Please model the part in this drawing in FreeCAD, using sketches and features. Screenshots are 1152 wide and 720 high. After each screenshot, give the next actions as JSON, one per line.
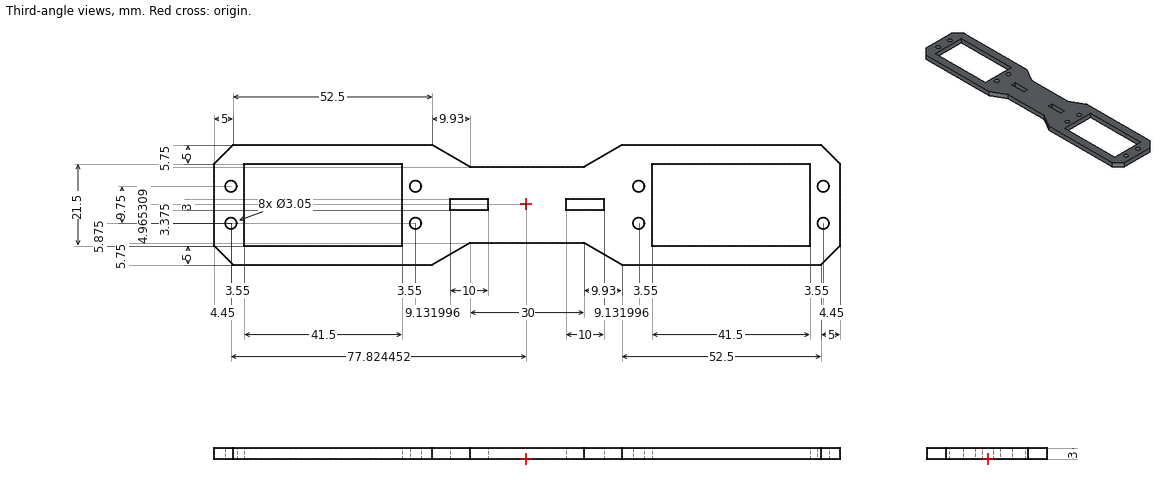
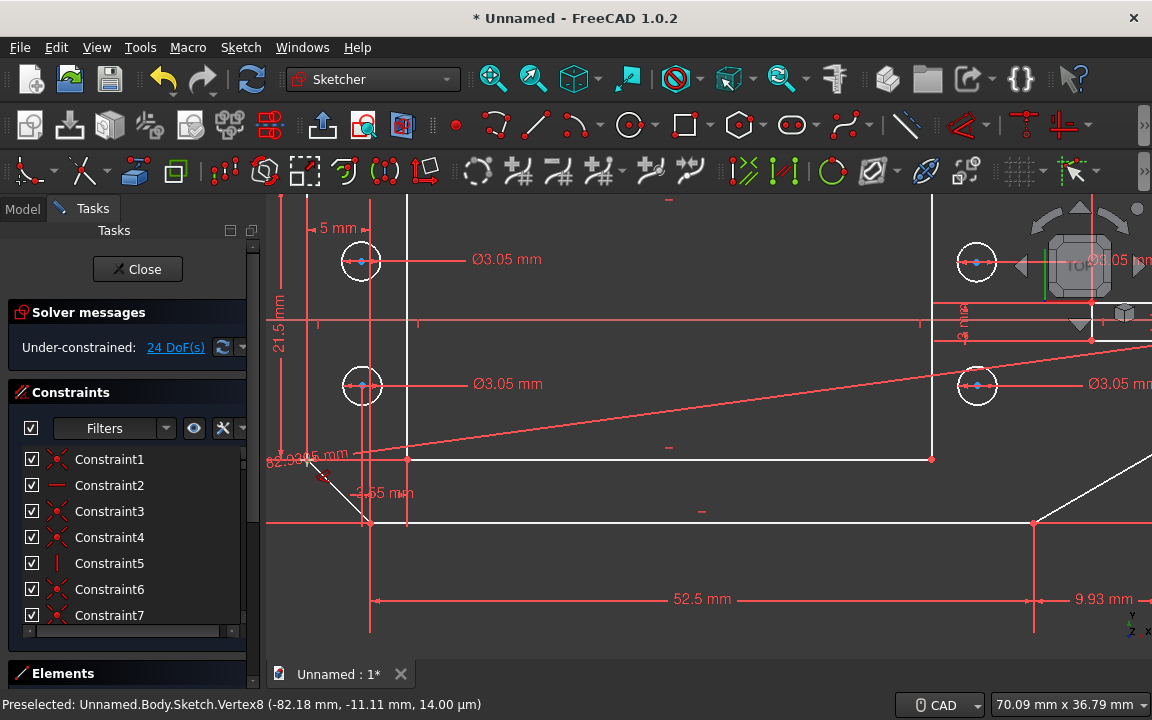
{"action": "left_click", "coordinate": [362, 386]}
{"action": "left_click", "coordinate": [335, 352]}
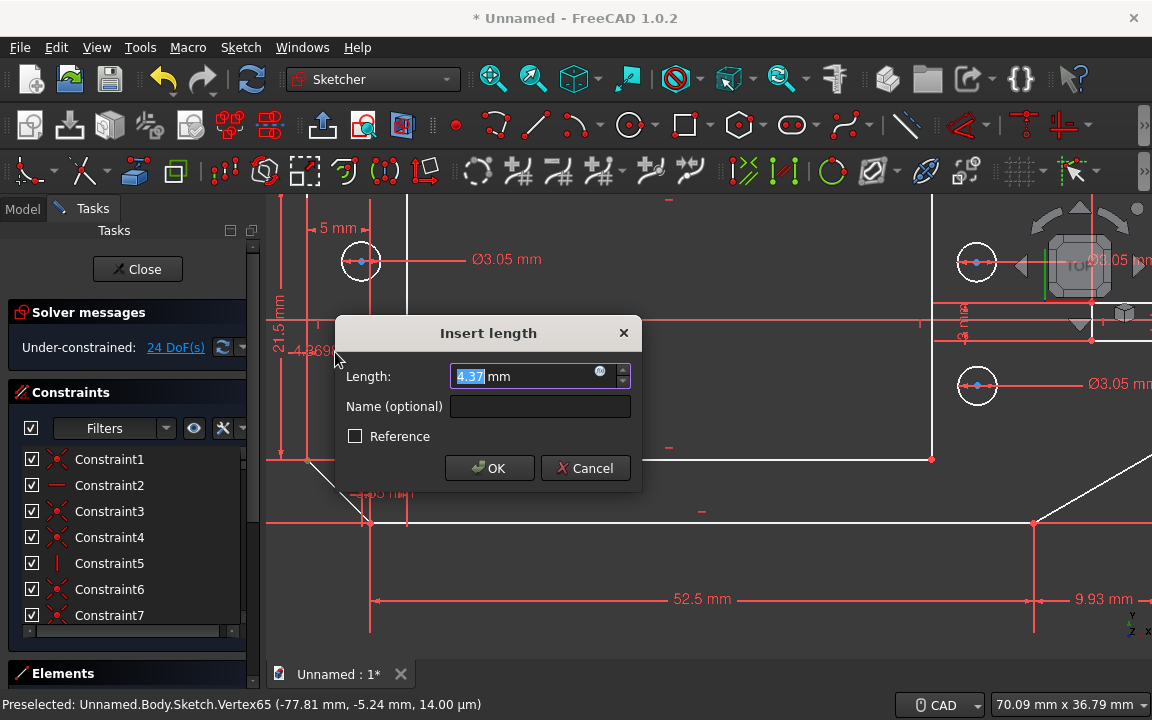
{"action": "type", "text": "4.45"}
{"action": "key", "text": "Return"}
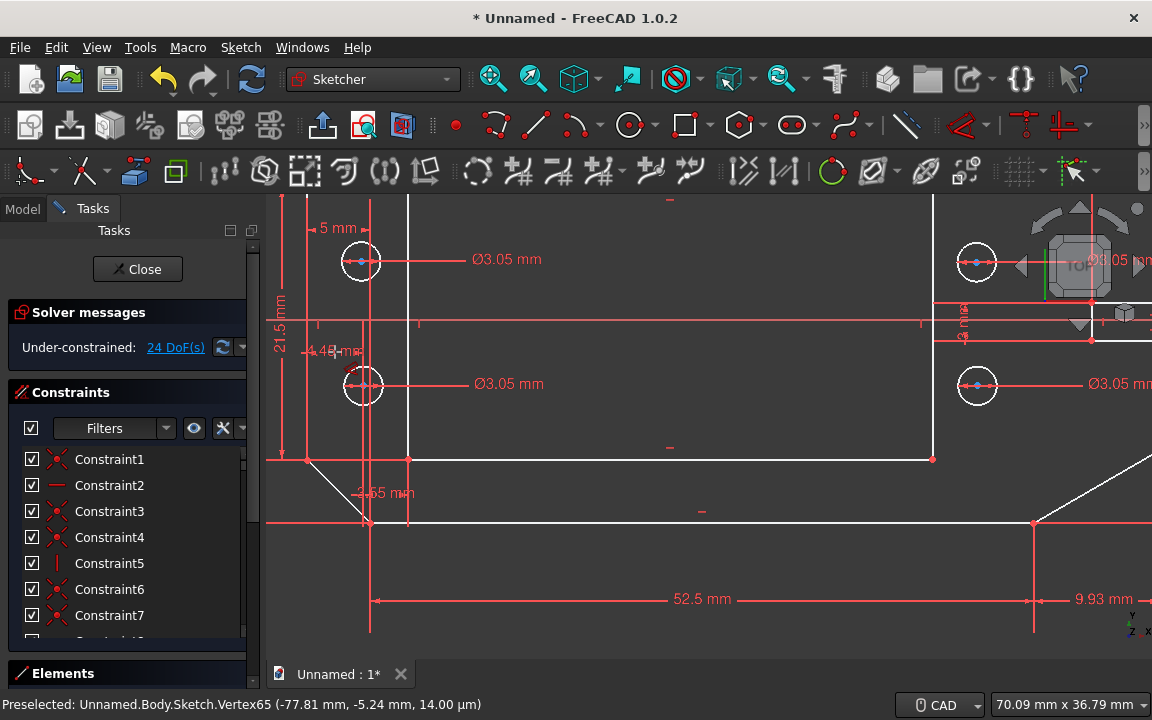
{"action": "left_click", "coordinate": [933, 460]}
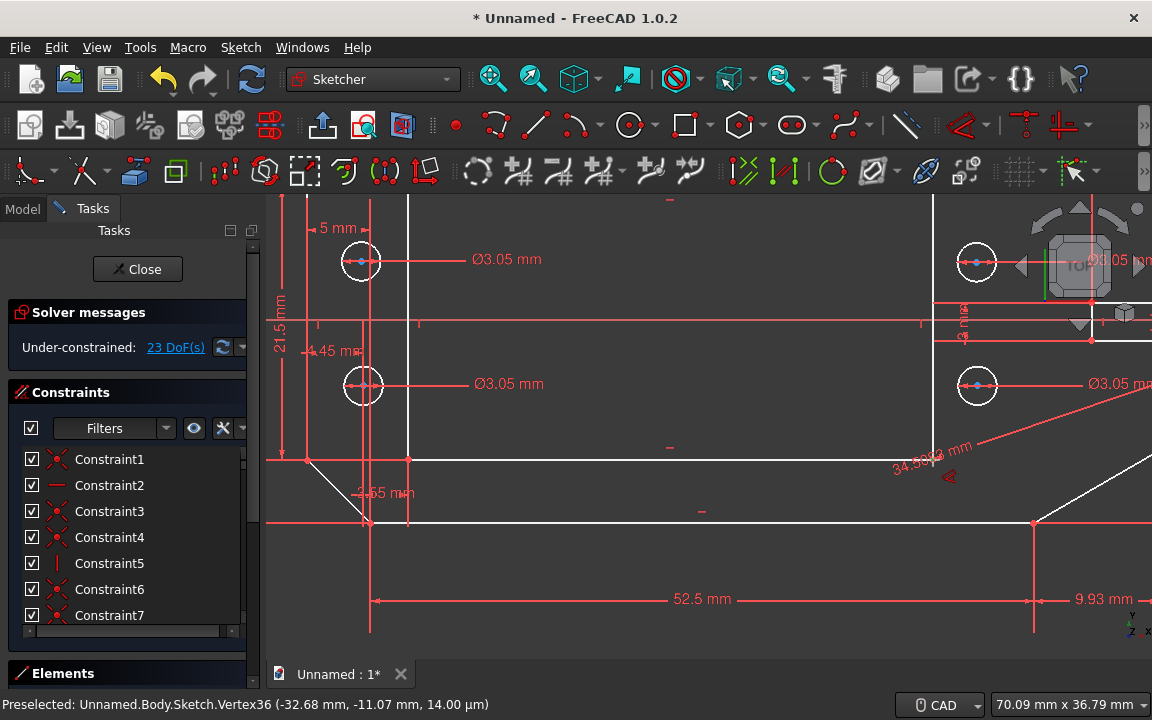
{"action": "left_click", "coordinate": [978, 386]}
{"action": "left_click", "coordinate": [955, 494]}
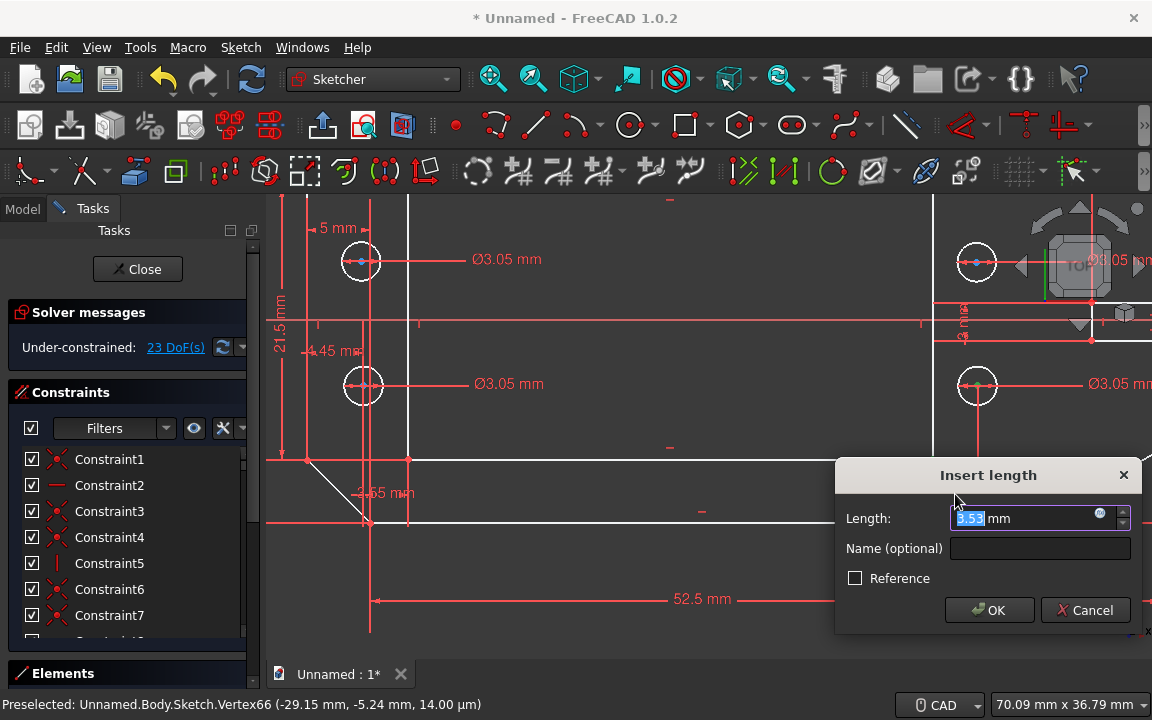
{"action": "type", "text": "3.55"}
{"action": "key", "text": "Return"}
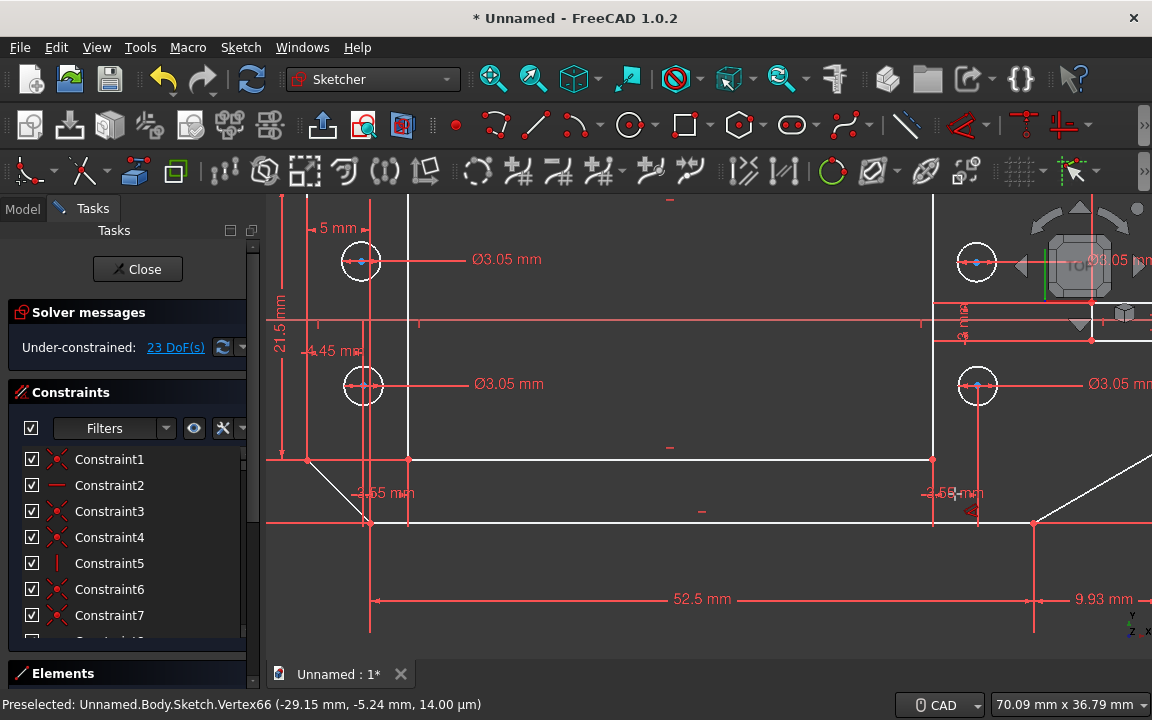
{"action": "scroll", "coordinate": [409, 461], "scroll_direction": "down", "scroll_amount": 7}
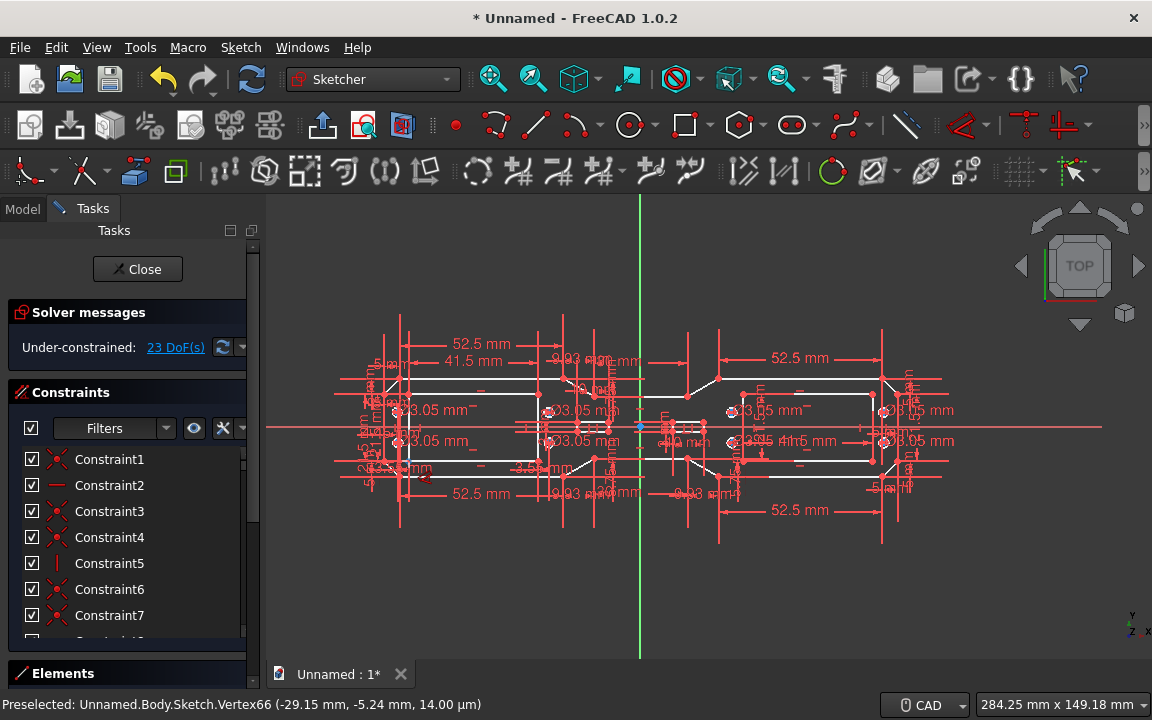
{"action": "scroll", "coordinate": [743, 461], "scroll_direction": "up", "scroll_amount": 7}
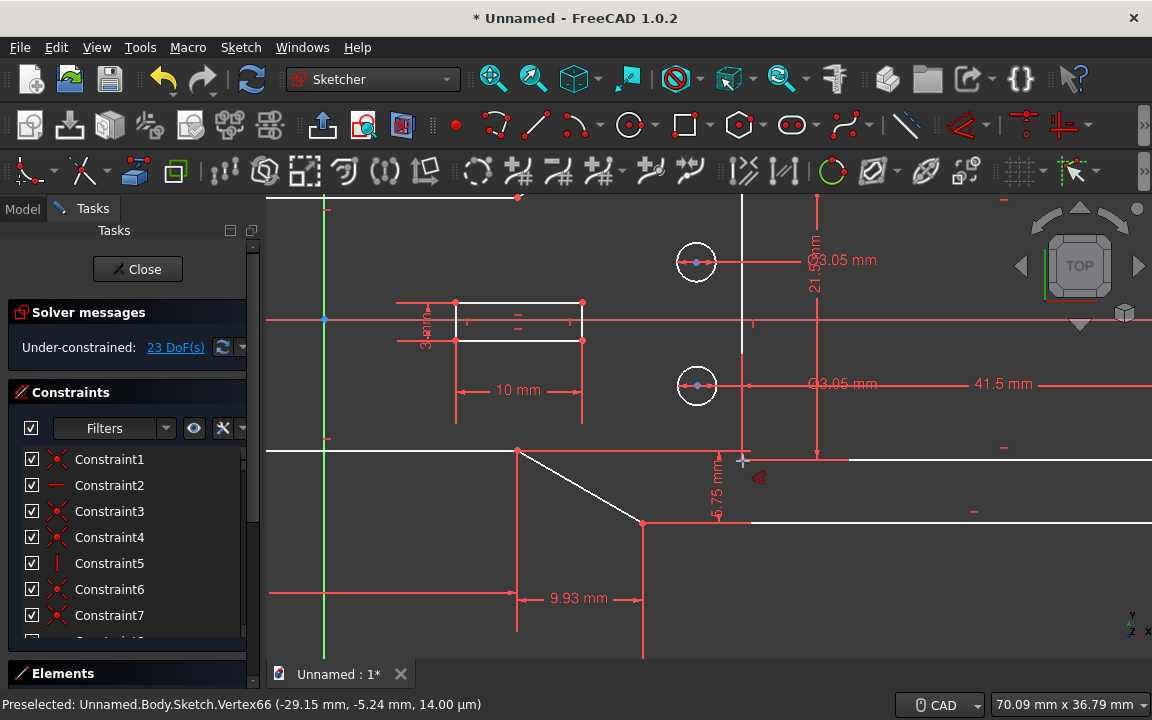
{"action": "left_click", "coordinate": [742, 460]}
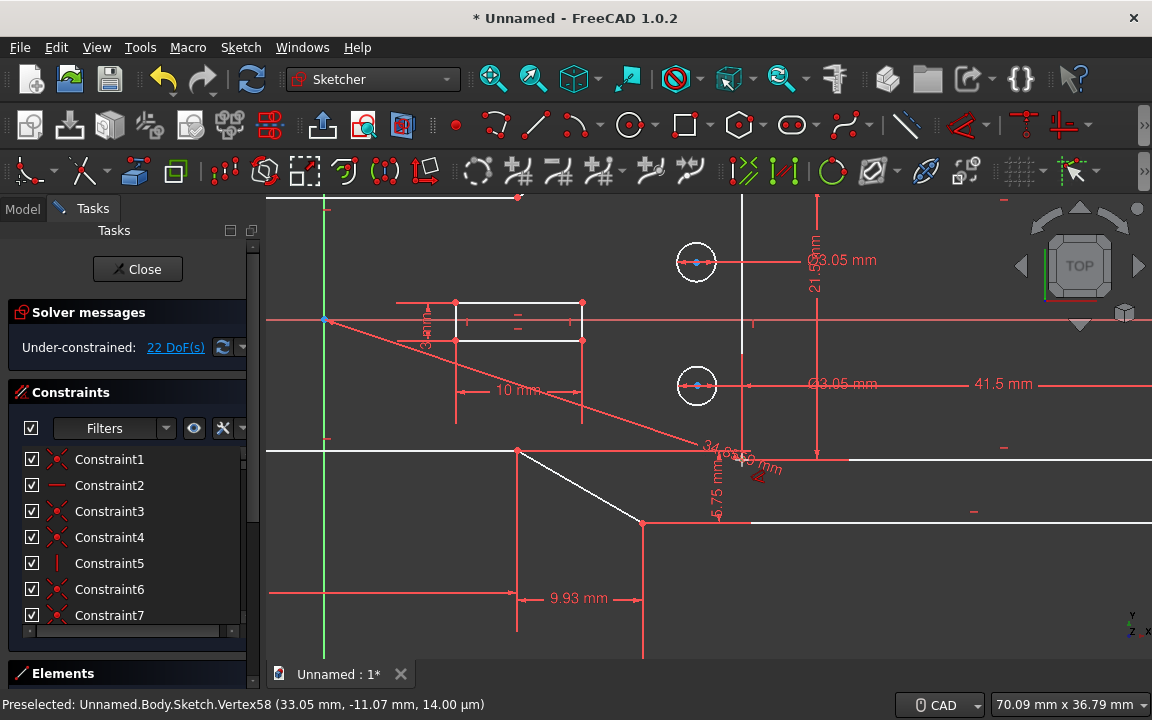
{"action": "left_click", "coordinate": [697, 386]}
{"action": "left_click", "coordinate": [720, 352]}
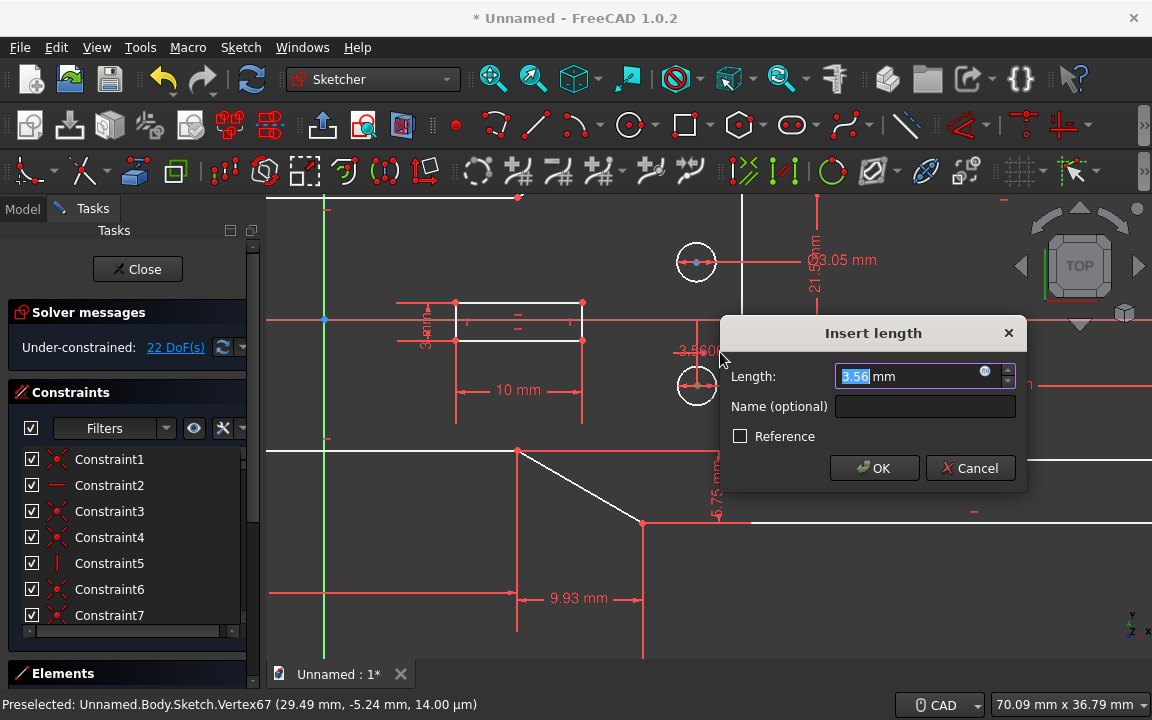
{"action": "type", "text": "3.55"}
{"action": "key", "text": "Return"}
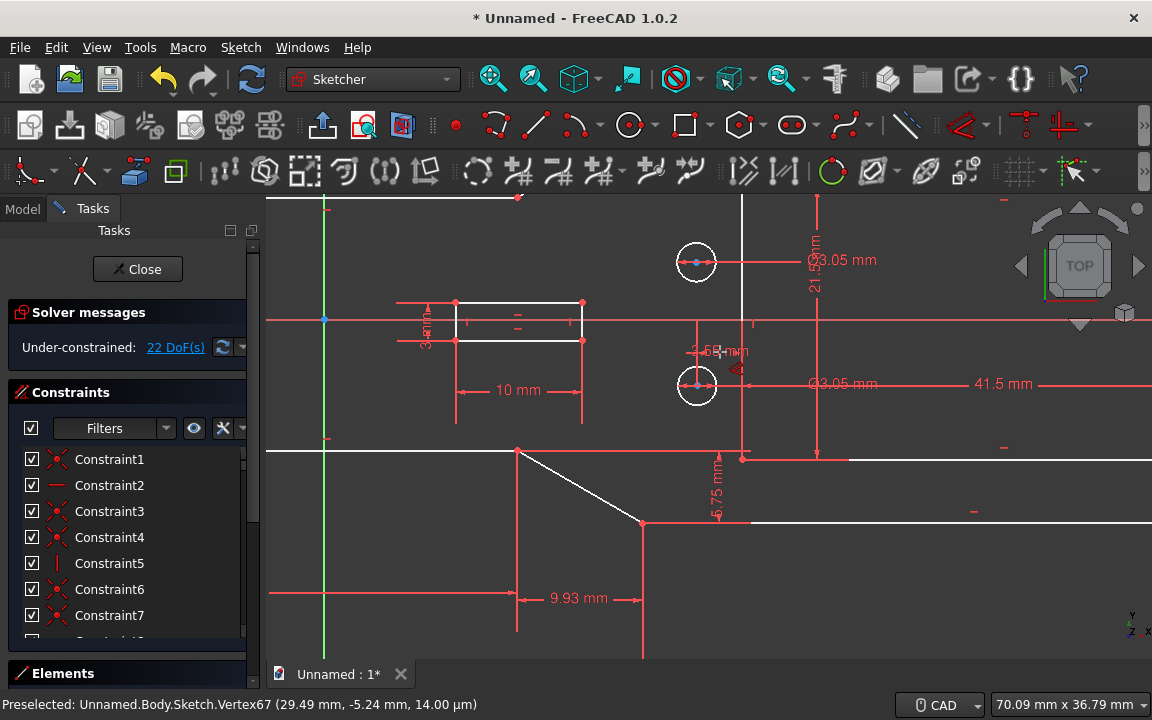
{"action": "scroll", "coordinate": [743, 461], "scroll_direction": "down", "scroll_amount": 7}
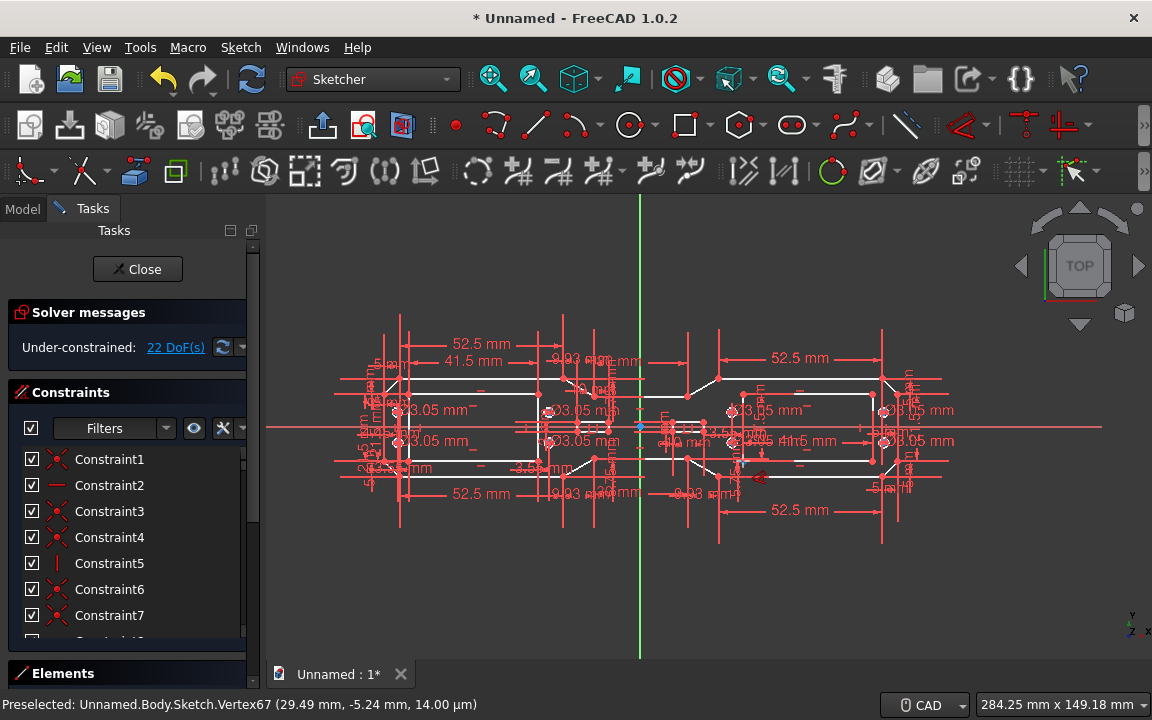
{"action": "scroll", "coordinate": [873, 461], "scroll_direction": "up", "scroll_amount": 7}